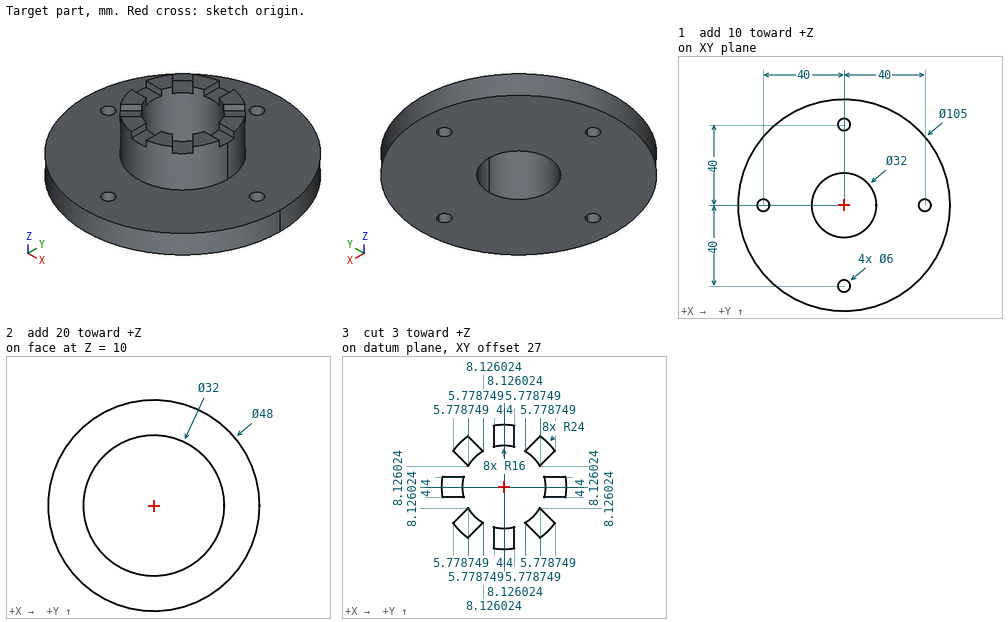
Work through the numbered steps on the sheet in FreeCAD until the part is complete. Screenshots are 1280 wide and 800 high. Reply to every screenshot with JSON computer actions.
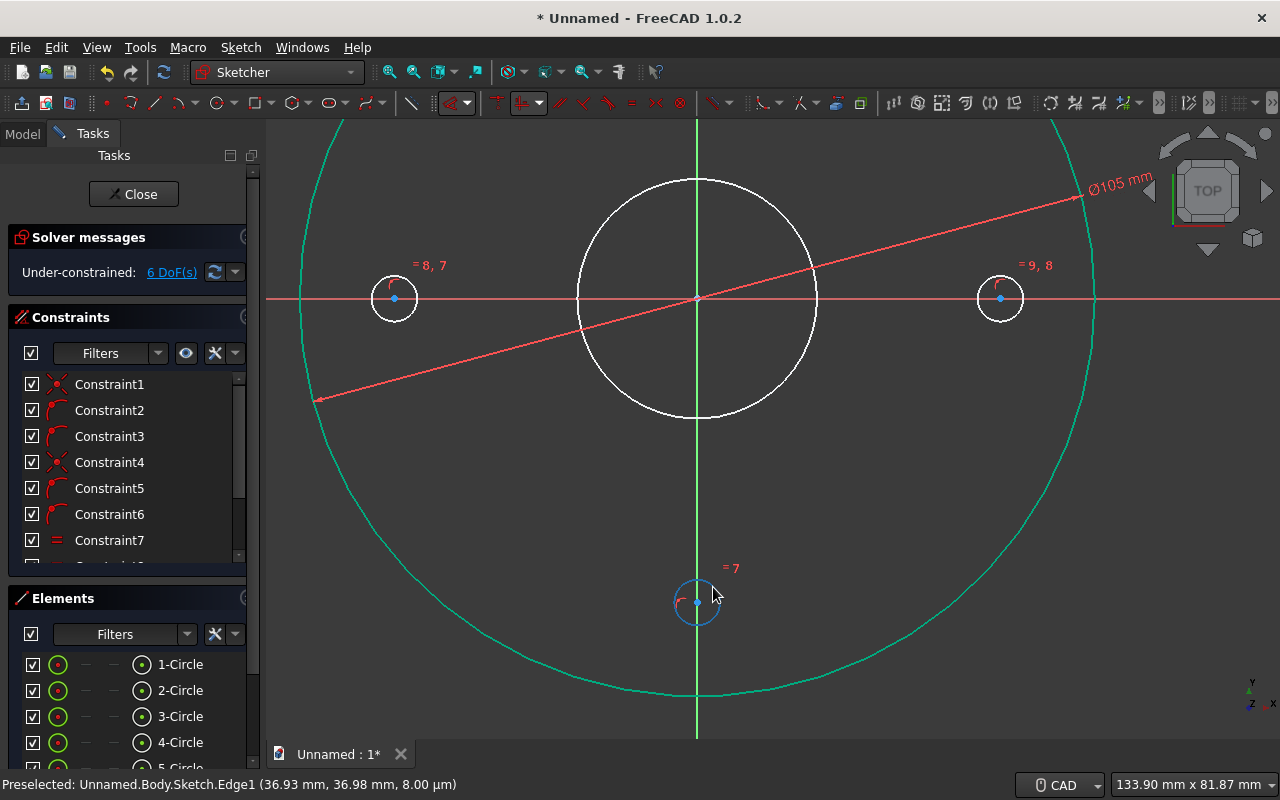
{"action": "left_click", "coordinate": [713, 586]}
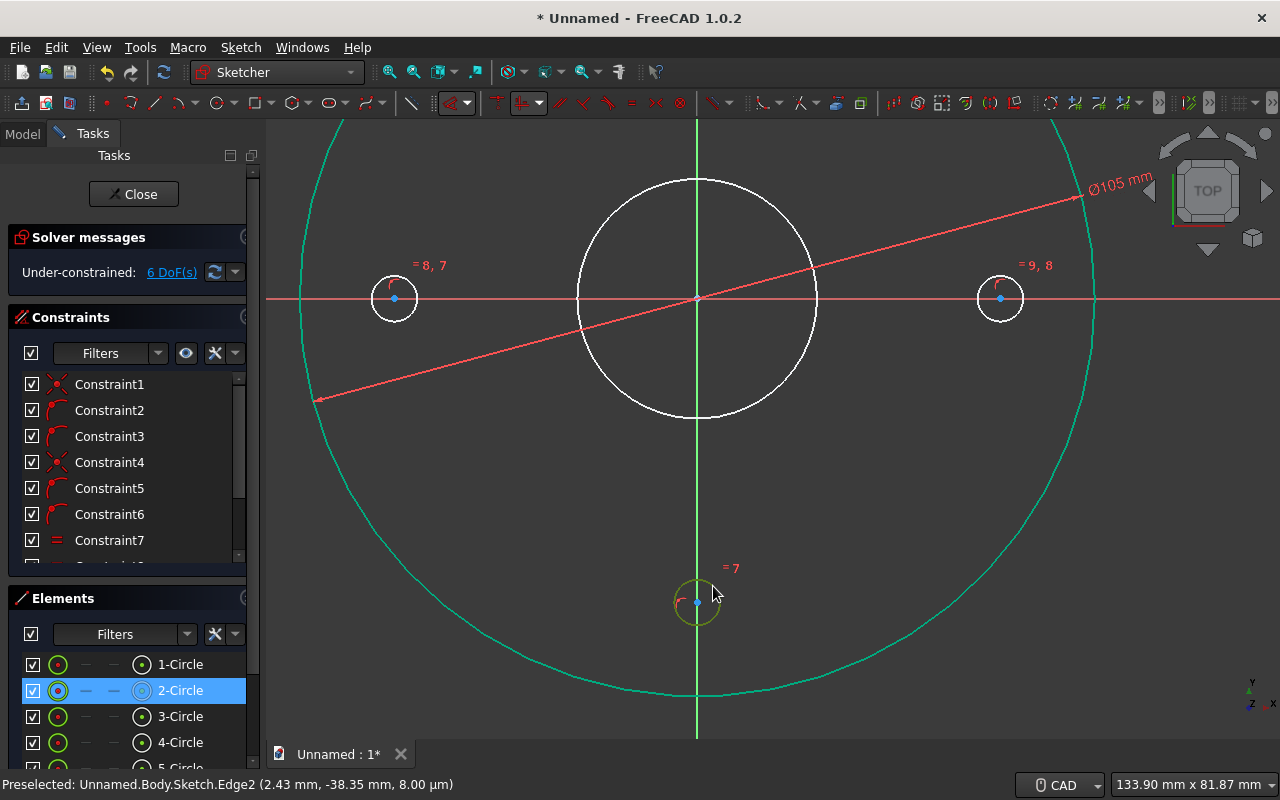
{"action": "key", "text": "k o"}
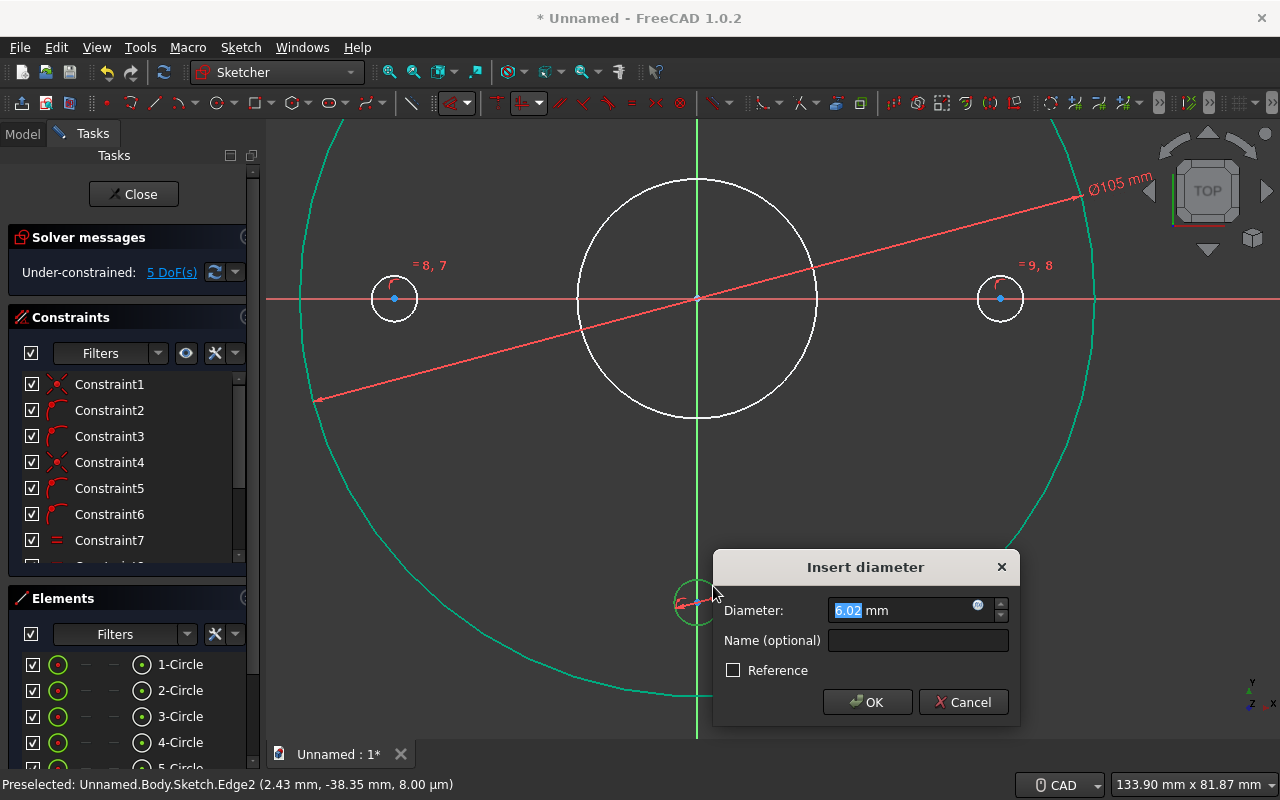
{"action": "type", "text": "6"}
{"action": "key", "text": "Return"}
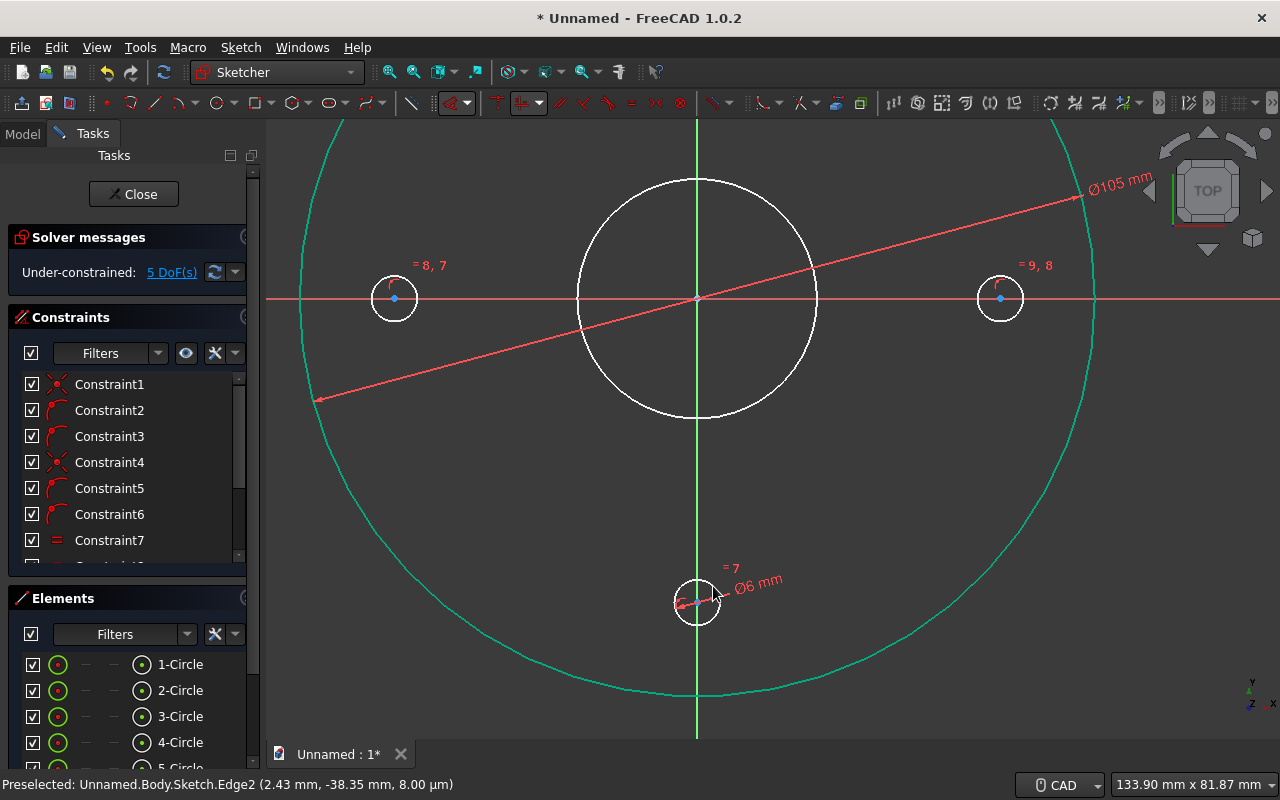
{"action": "left_click", "coordinate": [782, 214]}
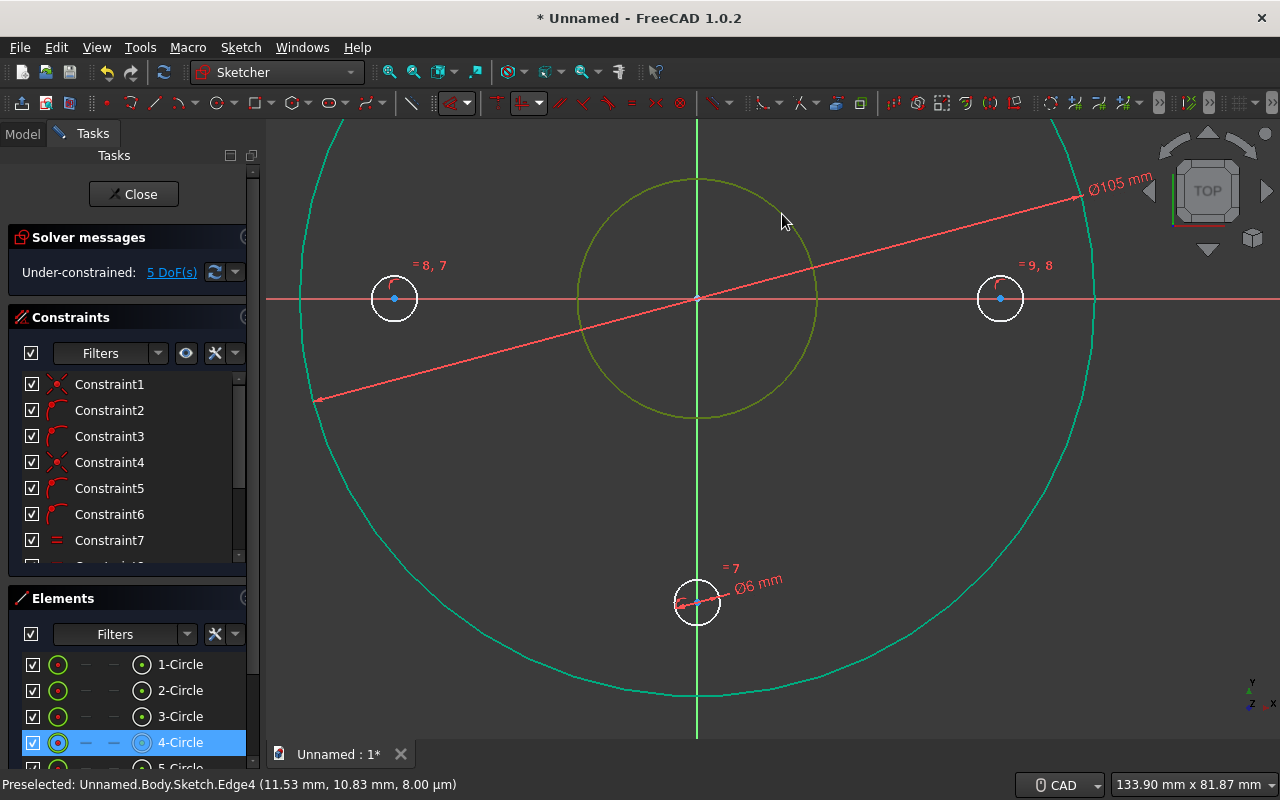
{"action": "left_click", "coordinate": [470, 104]}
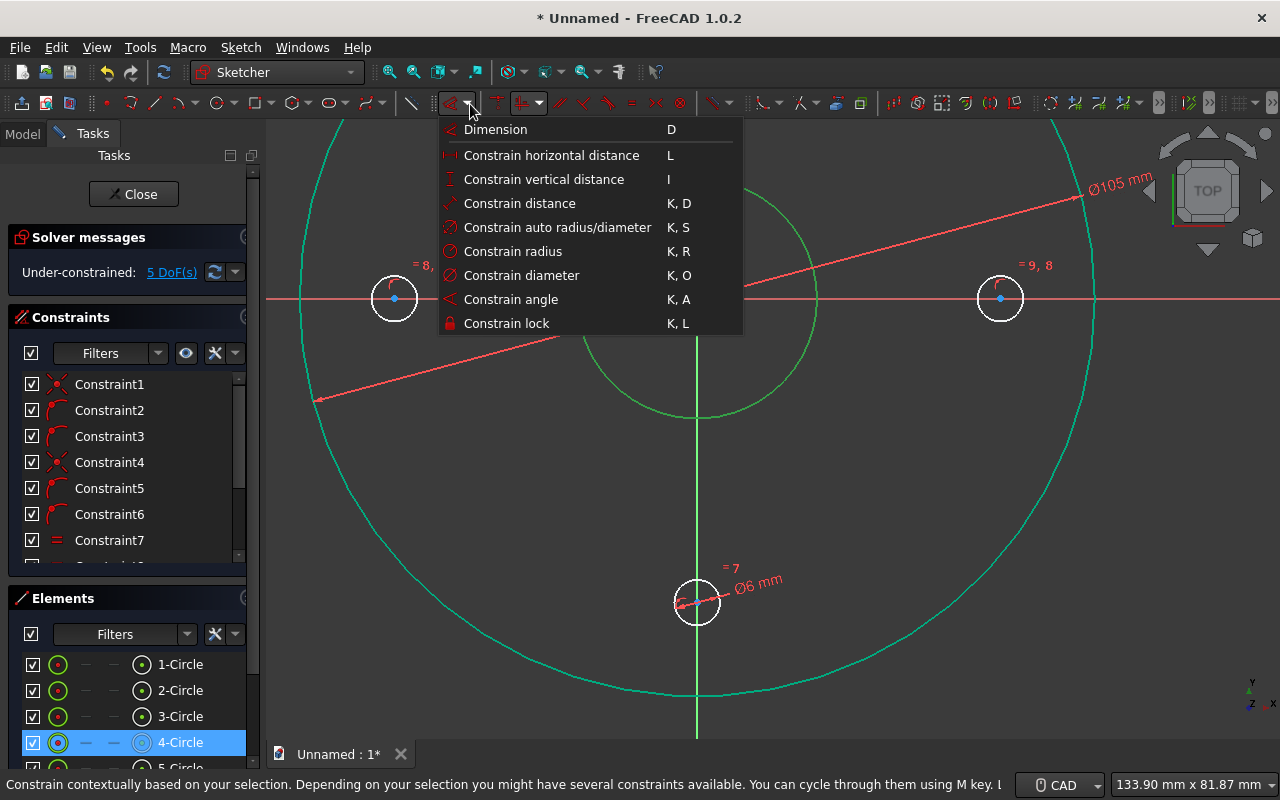
{"action": "left_click", "coordinate": [591, 275]}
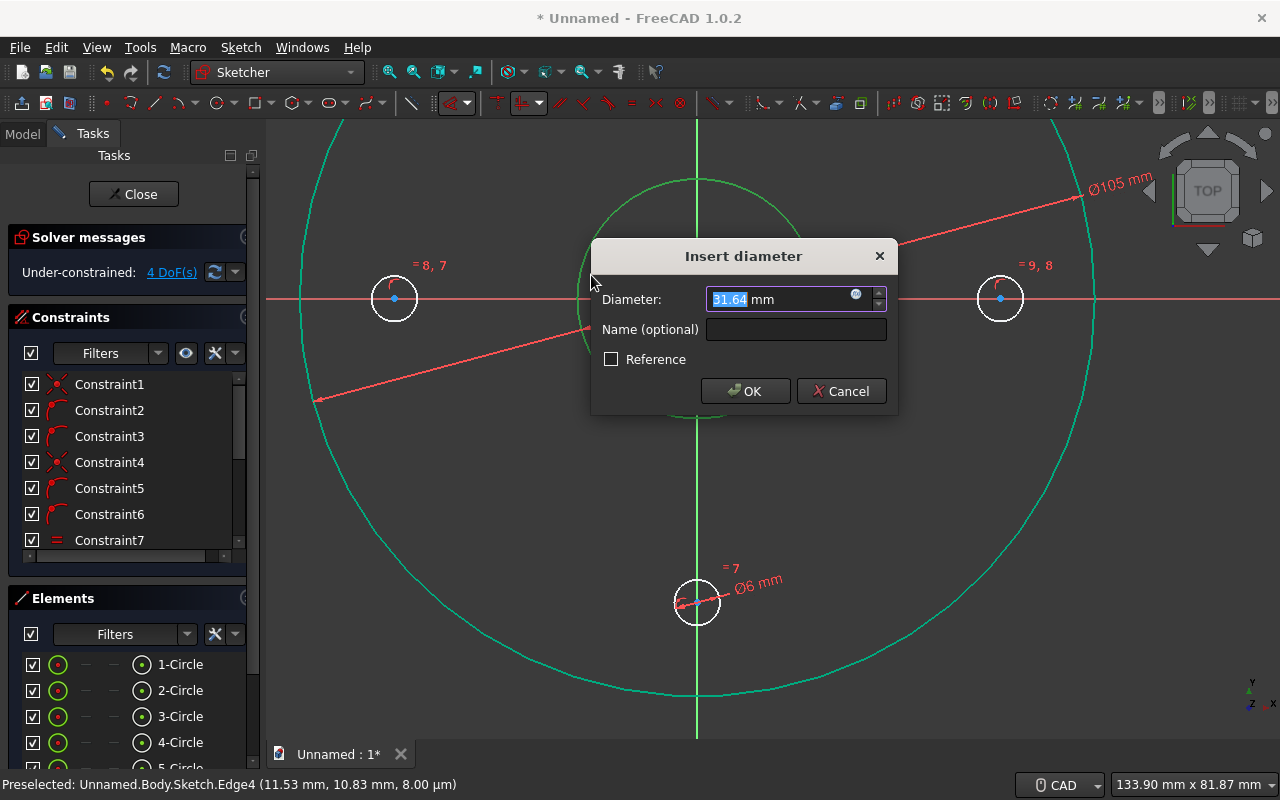
{"action": "type", "text": "32"}
{"action": "key", "text": "Return"}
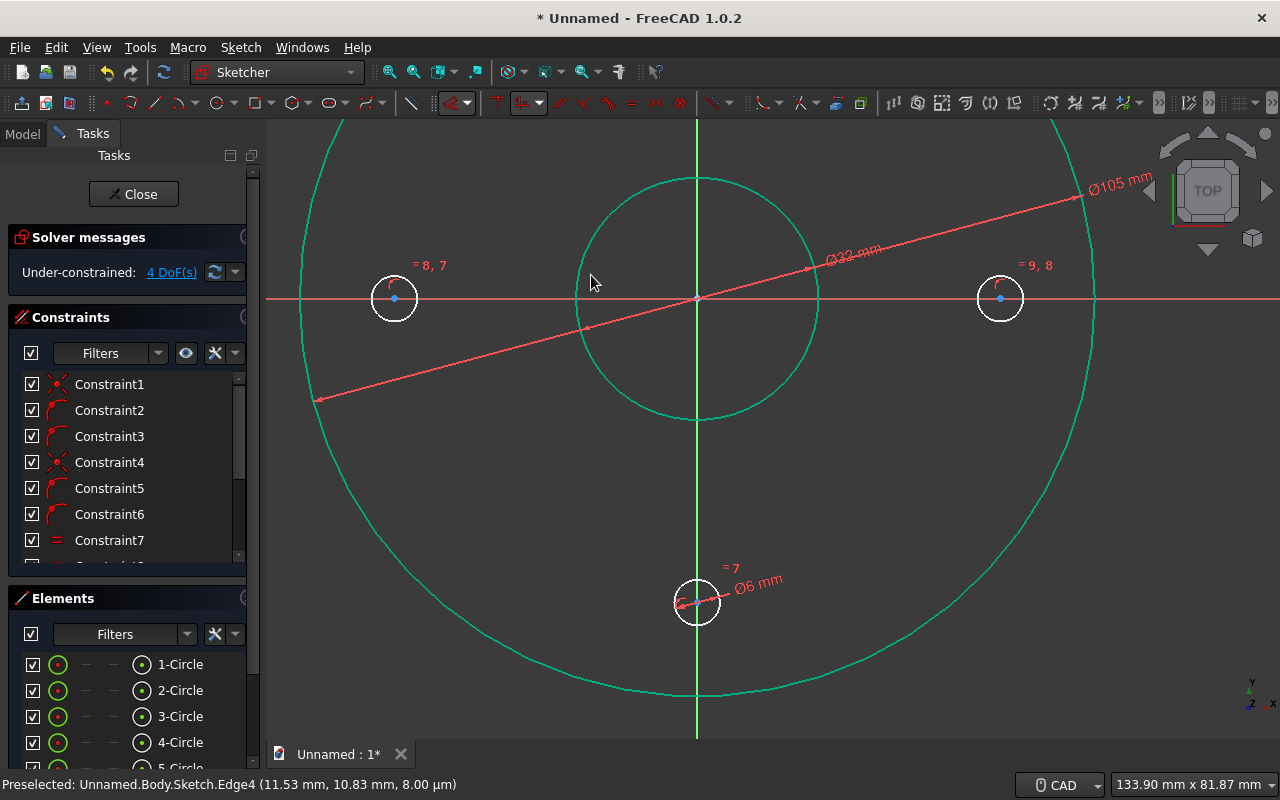
{"action": "left_click", "coordinate": [697, 603]}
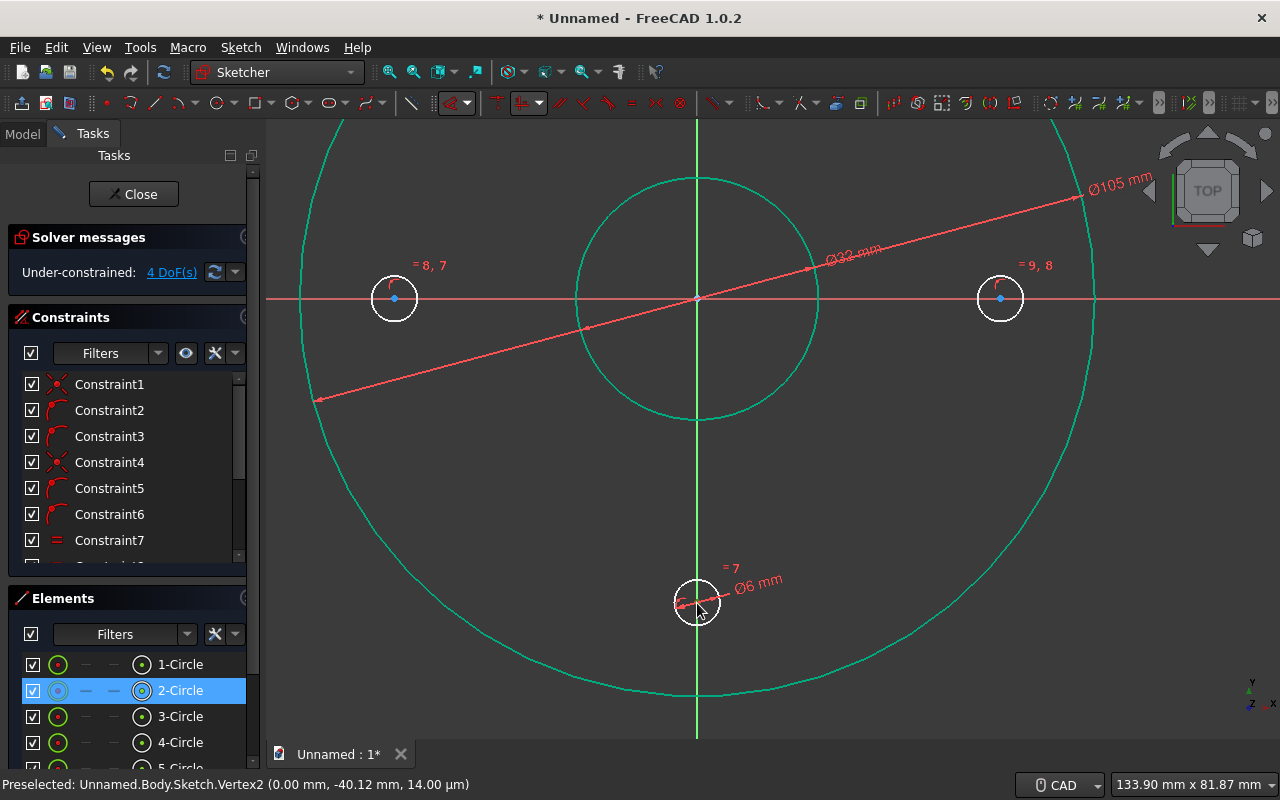
{"action": "left_click", "coordinate": [470, 104]}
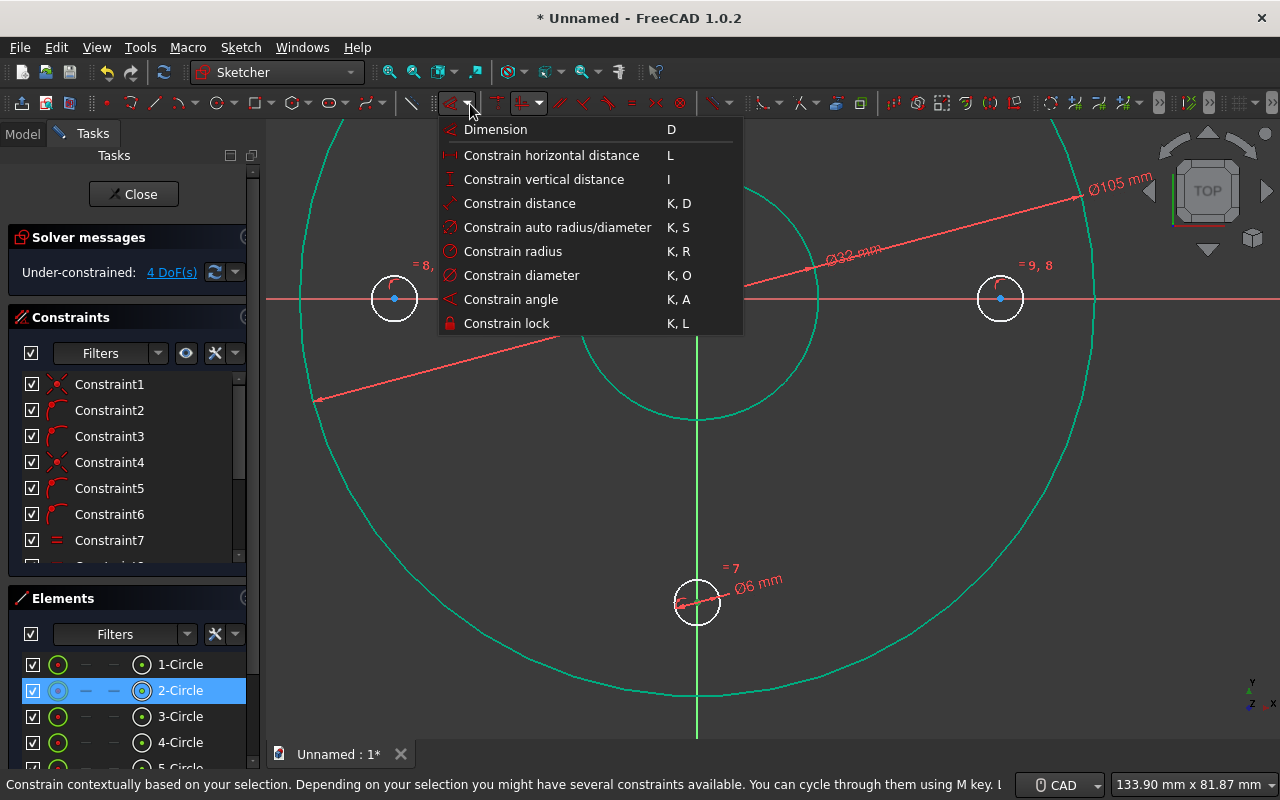
{"action": "left_click", "coordinate": [591, 179]}